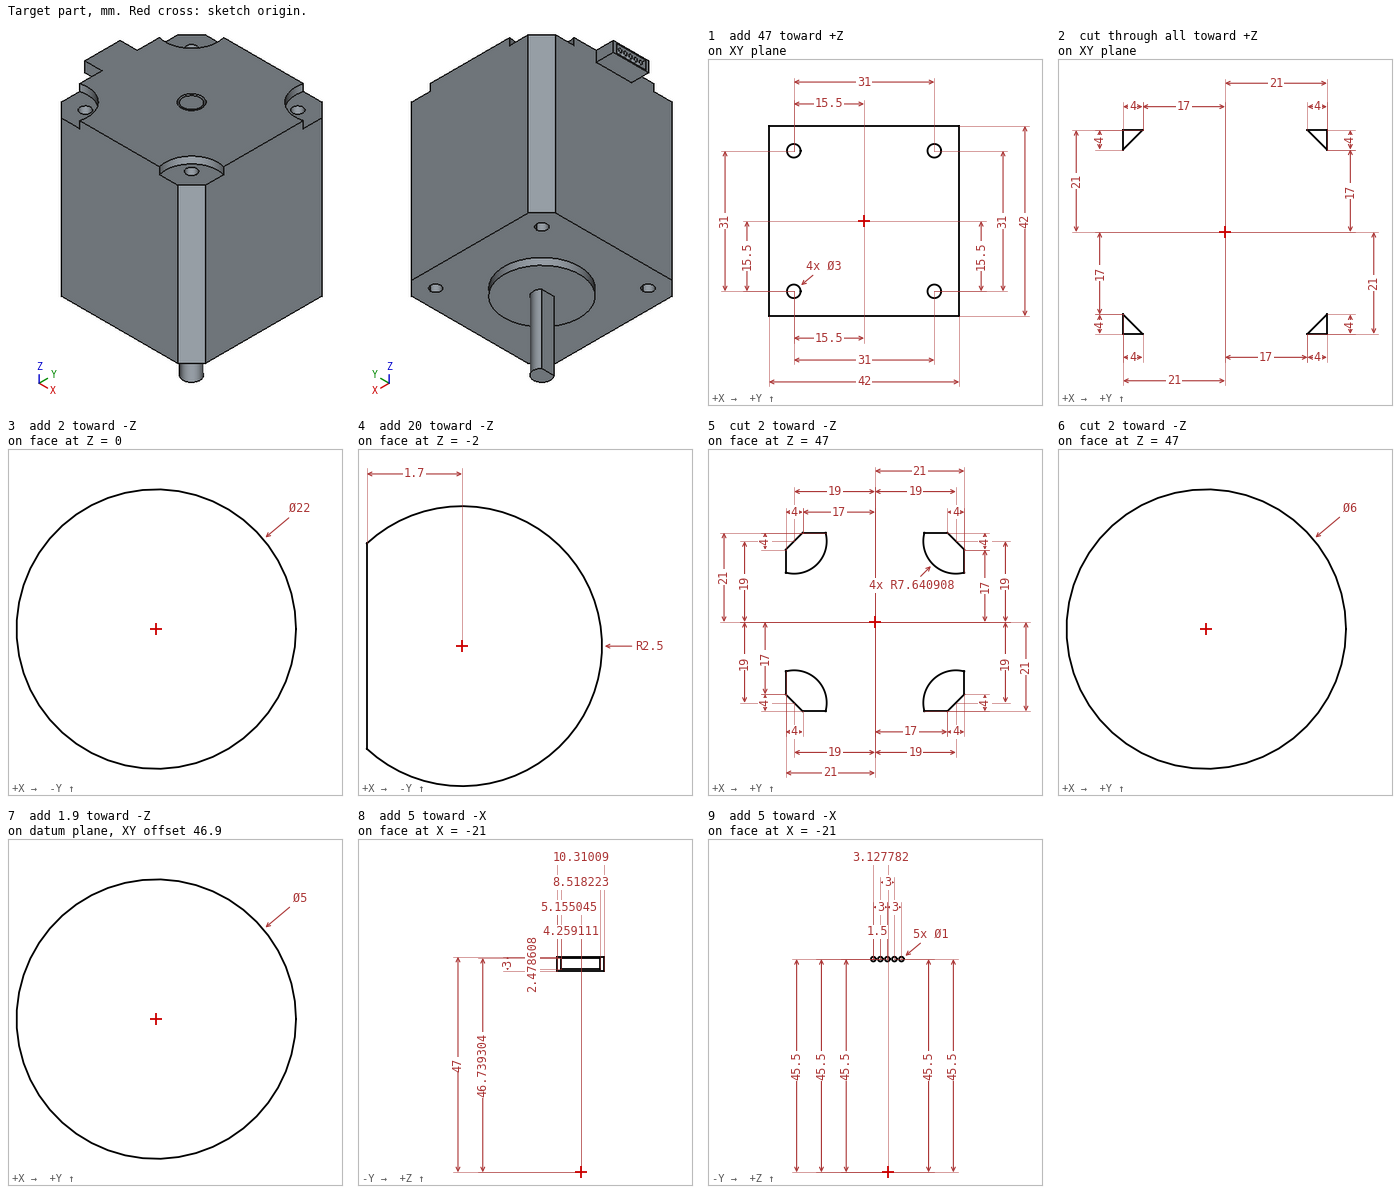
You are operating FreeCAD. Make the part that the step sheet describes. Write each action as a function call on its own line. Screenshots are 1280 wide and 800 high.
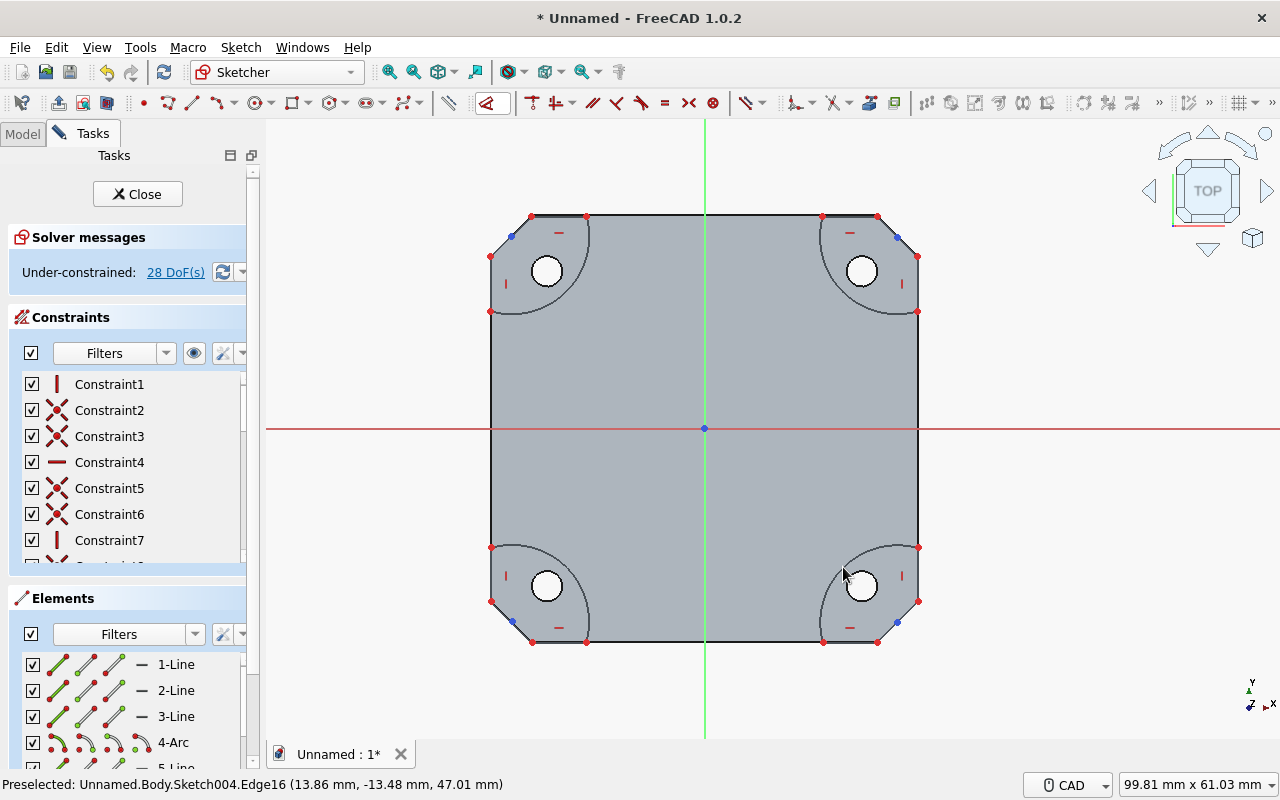
click(825, 265)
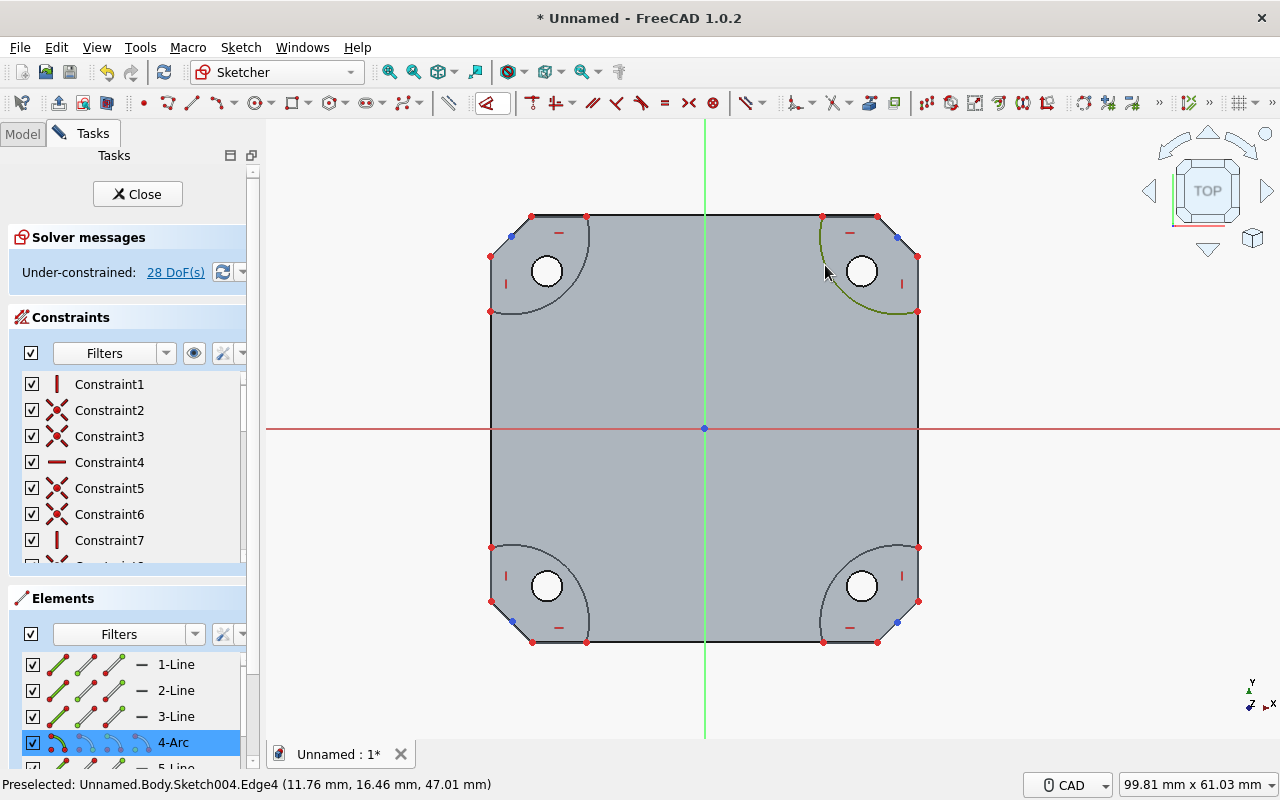
click(584, 595)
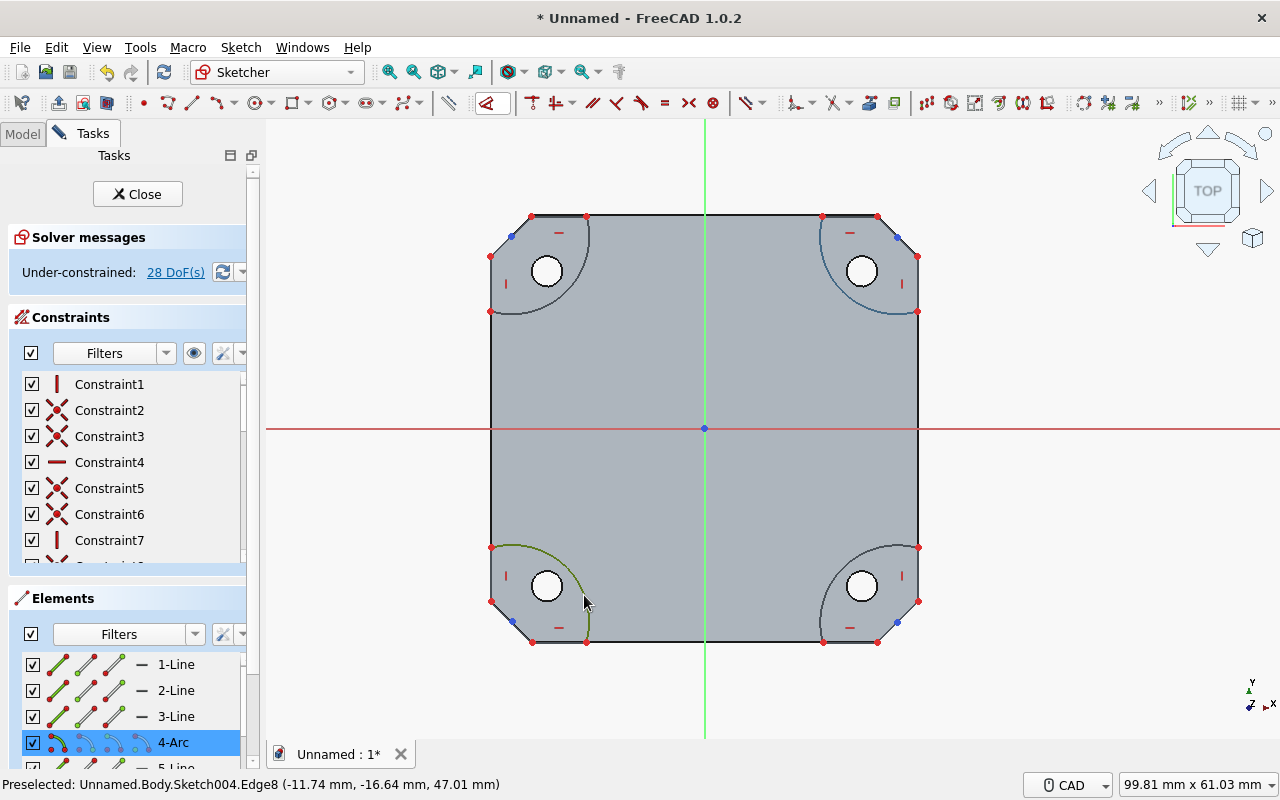
click(539, 309)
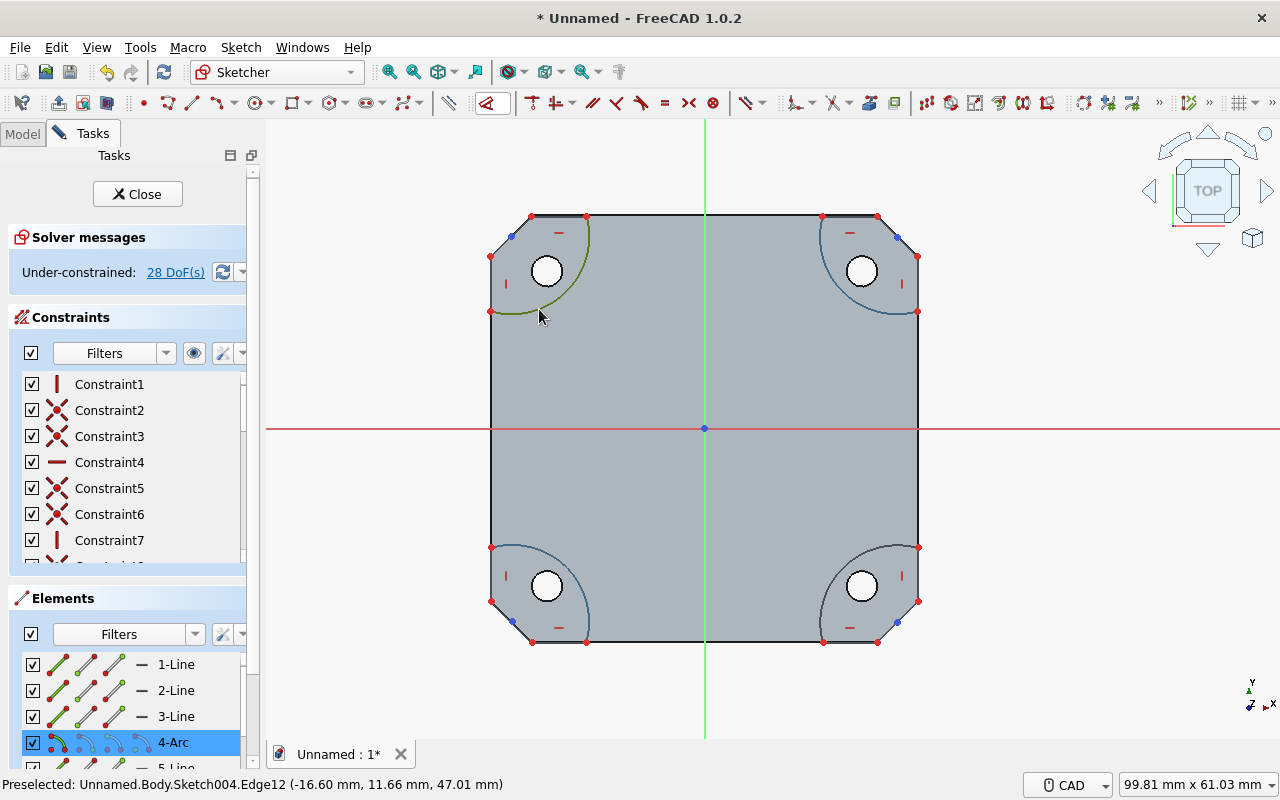
click(870, 550)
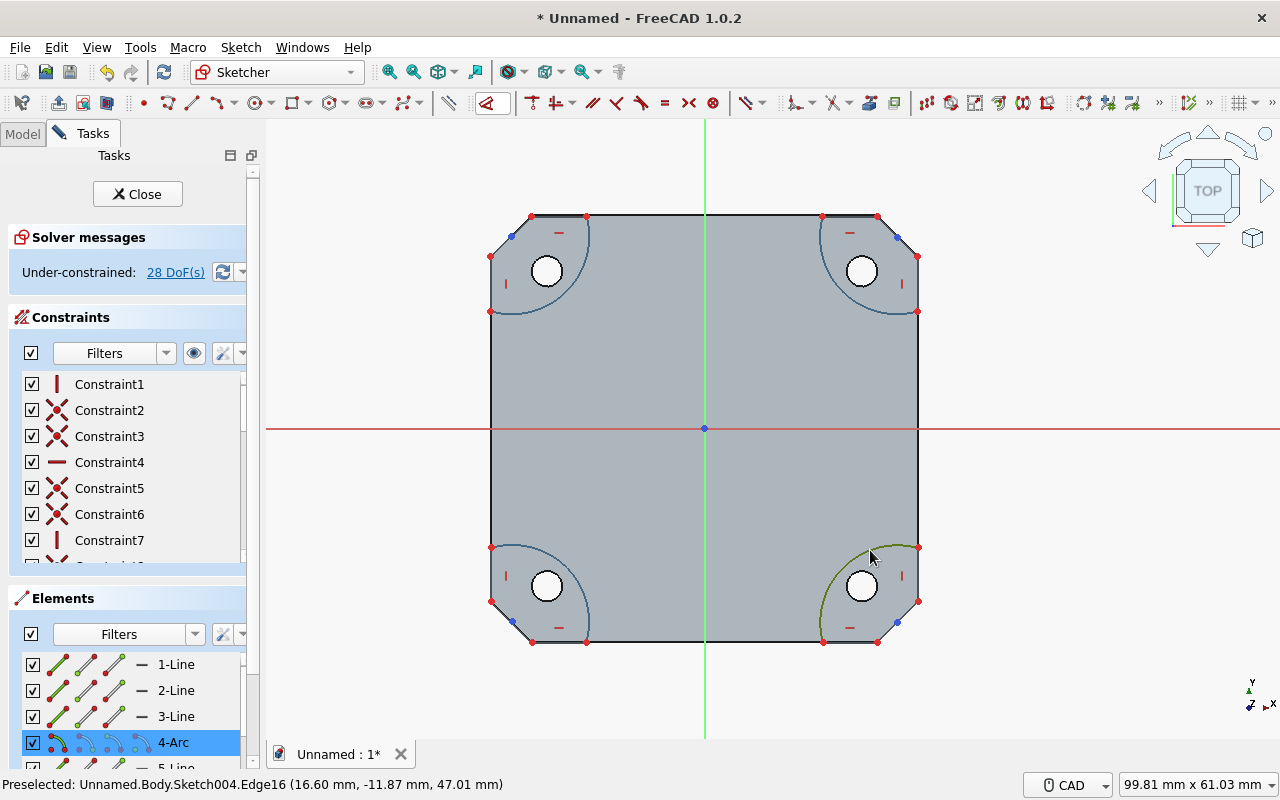
click(666, 104)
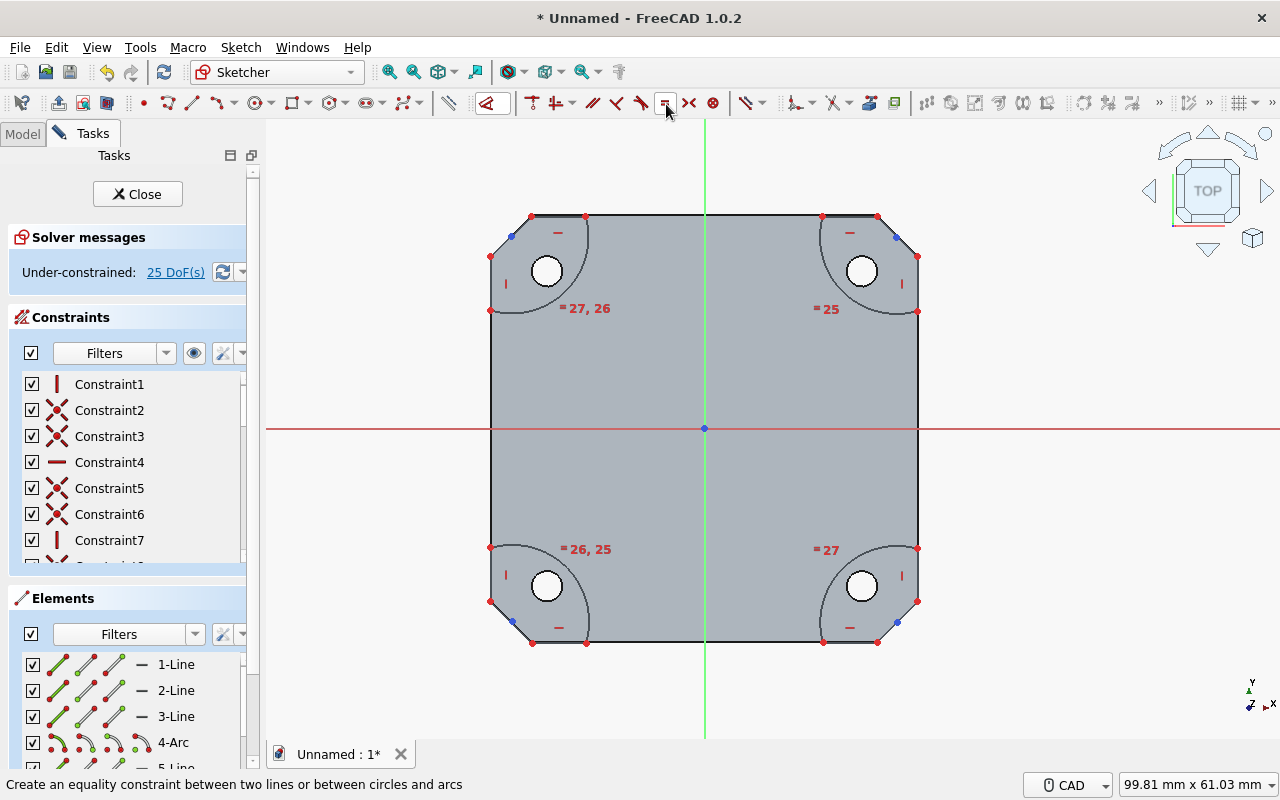
click(825, 265)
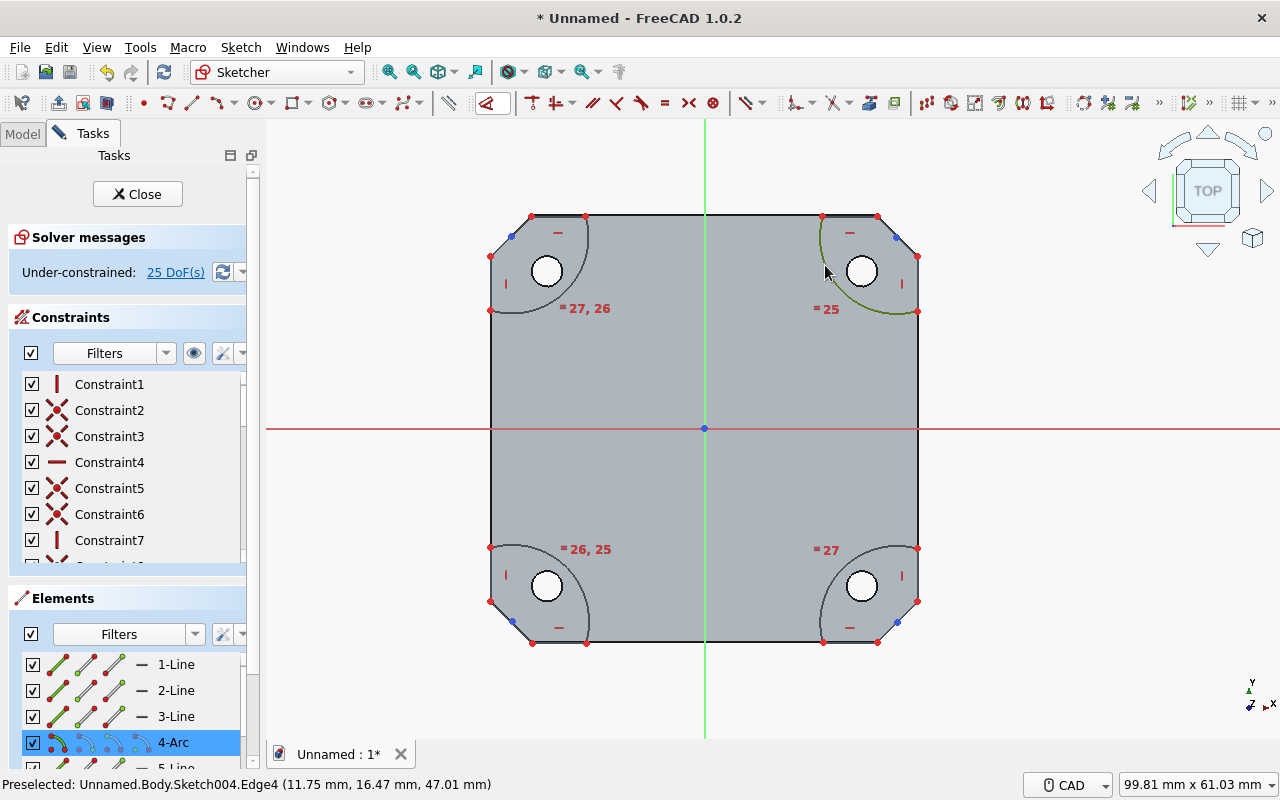
key(k)
key(r)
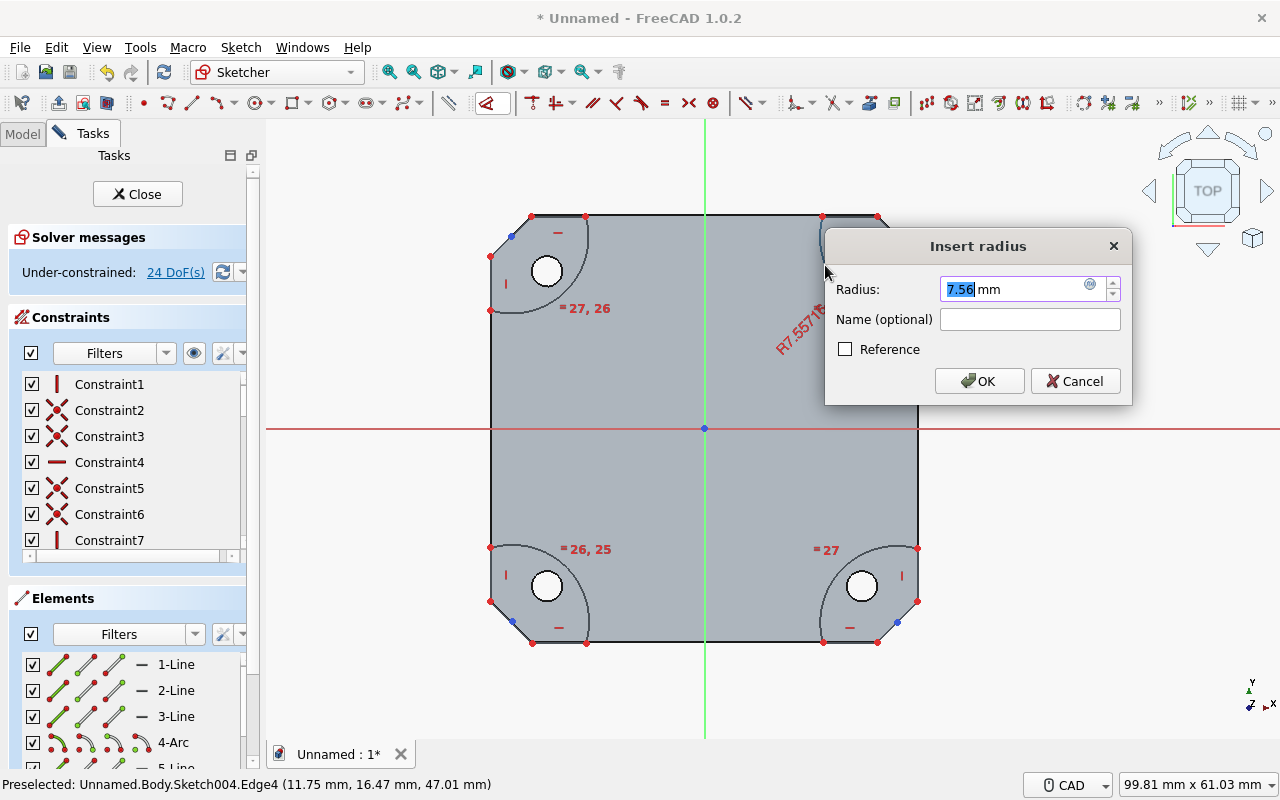
text(7.640908)
key(Return)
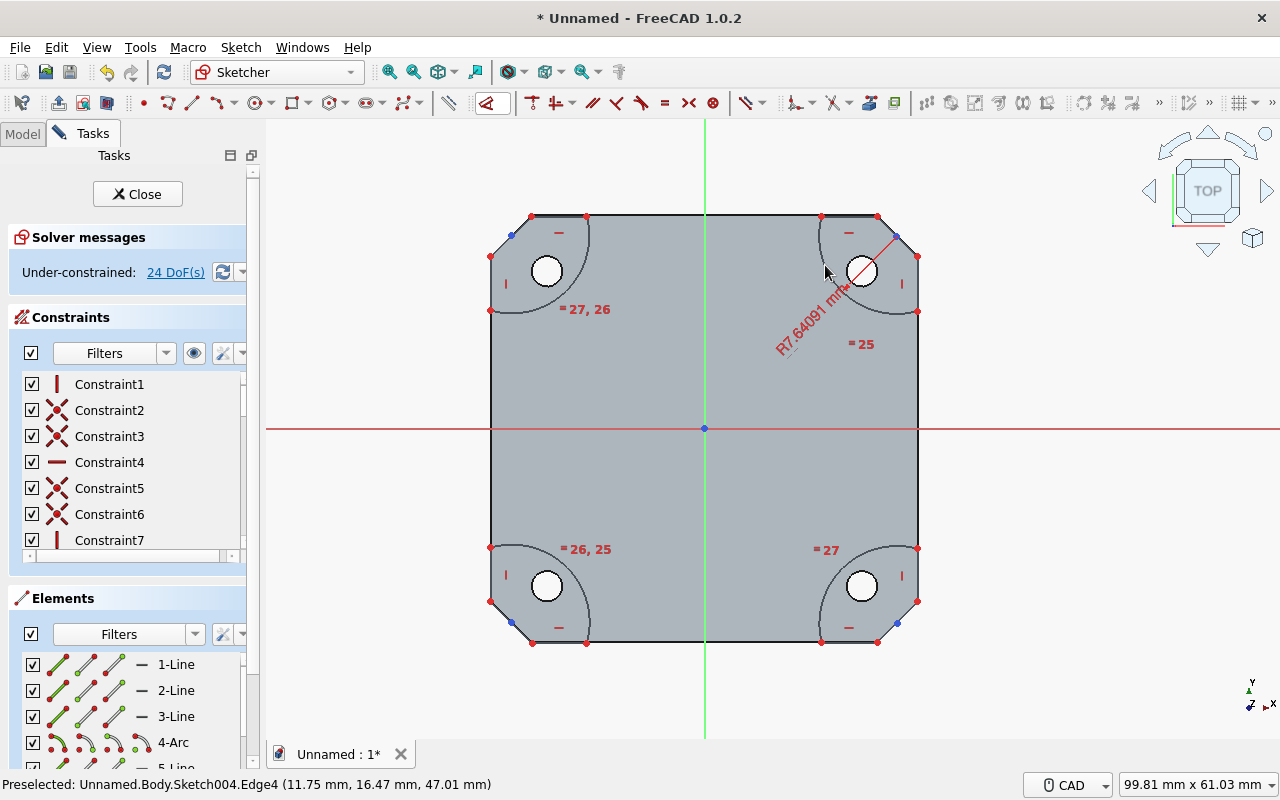
click(906, 245)